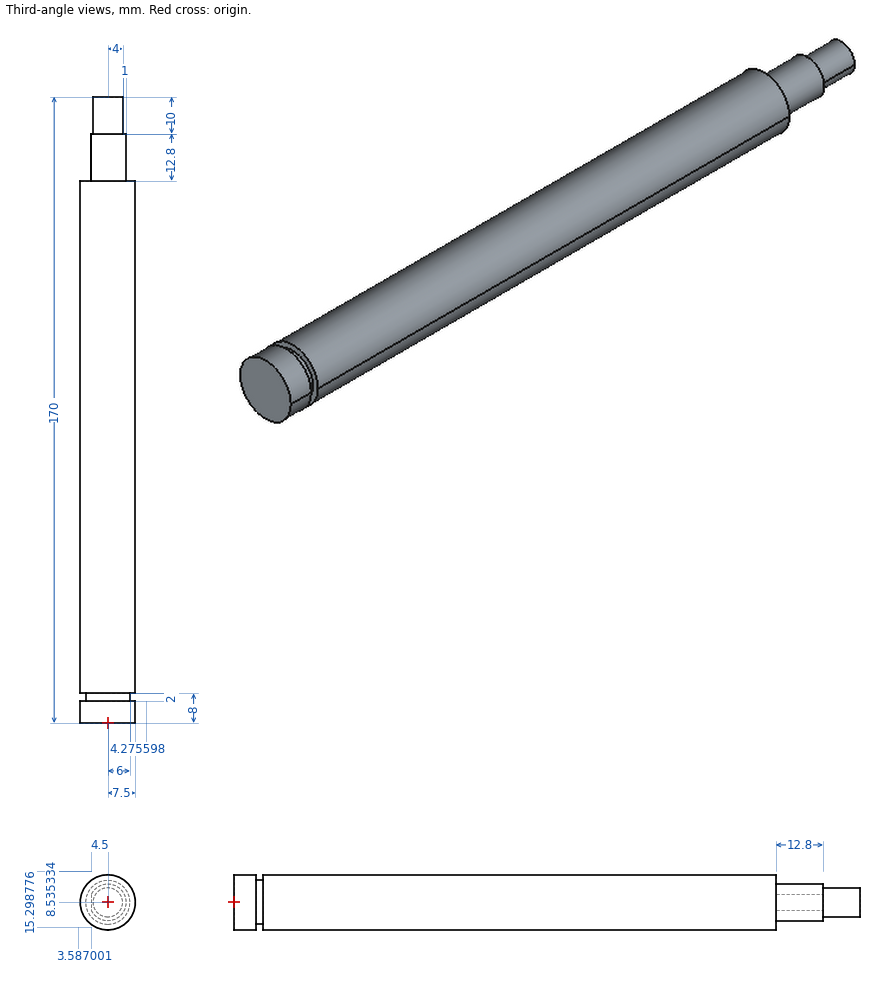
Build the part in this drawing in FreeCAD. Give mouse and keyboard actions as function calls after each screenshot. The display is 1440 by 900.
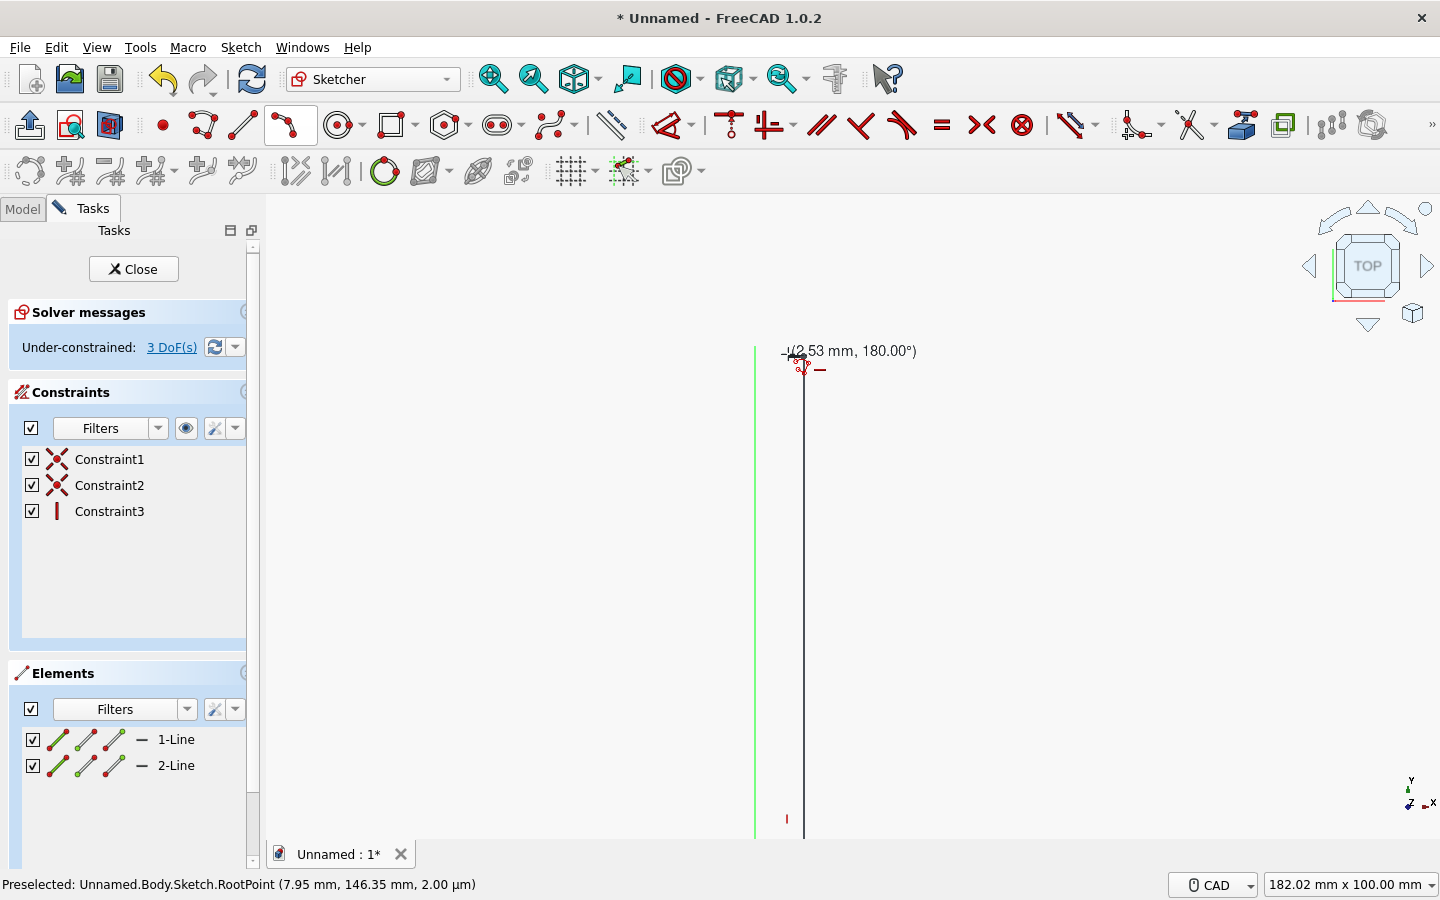
click(787, 354)
click(787, 271)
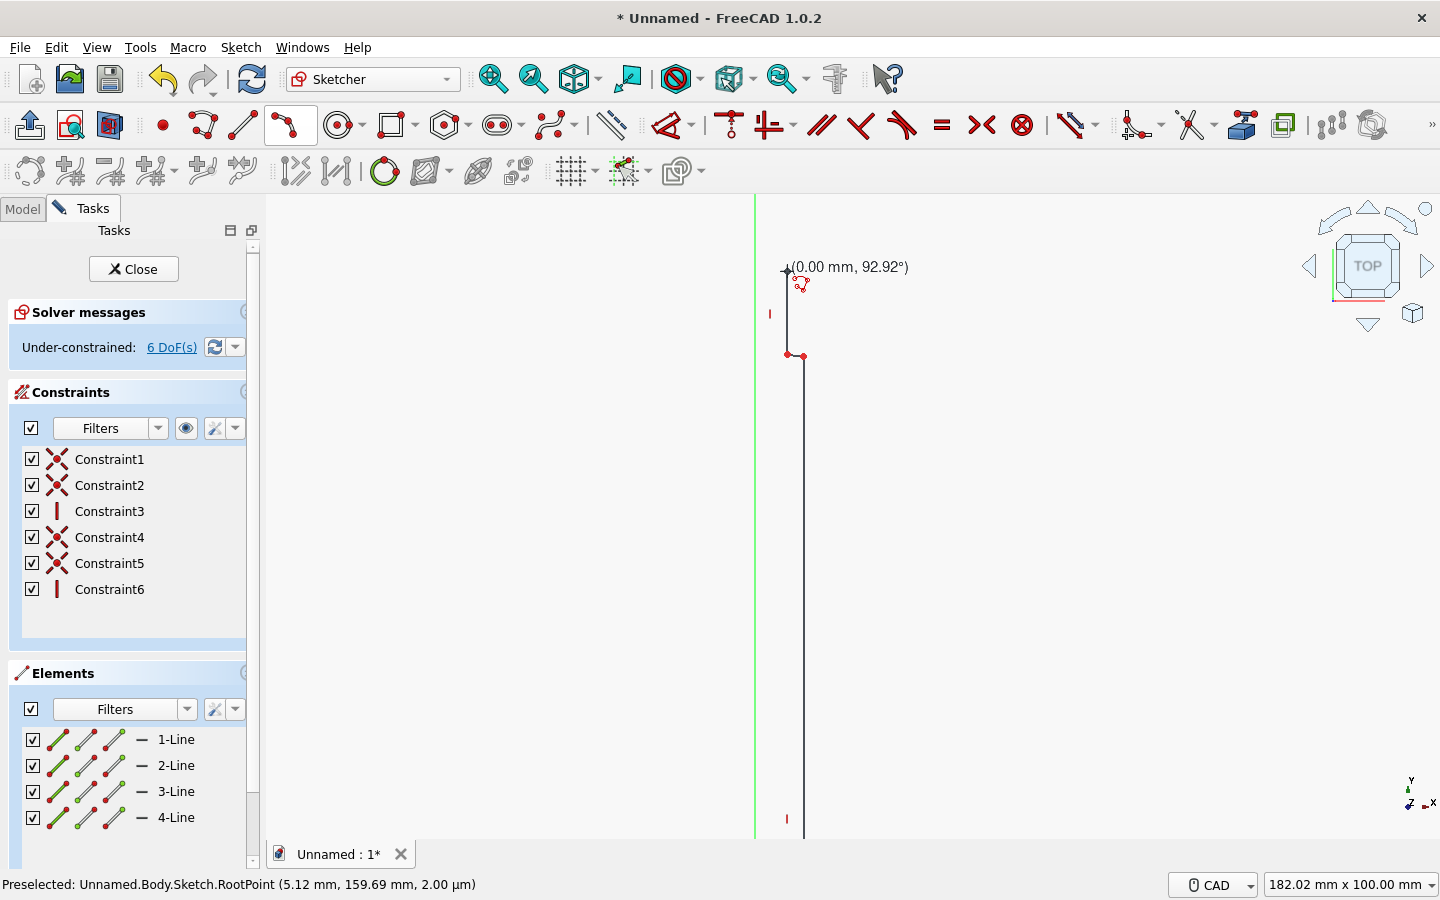
scroll(781, 271, up, 5)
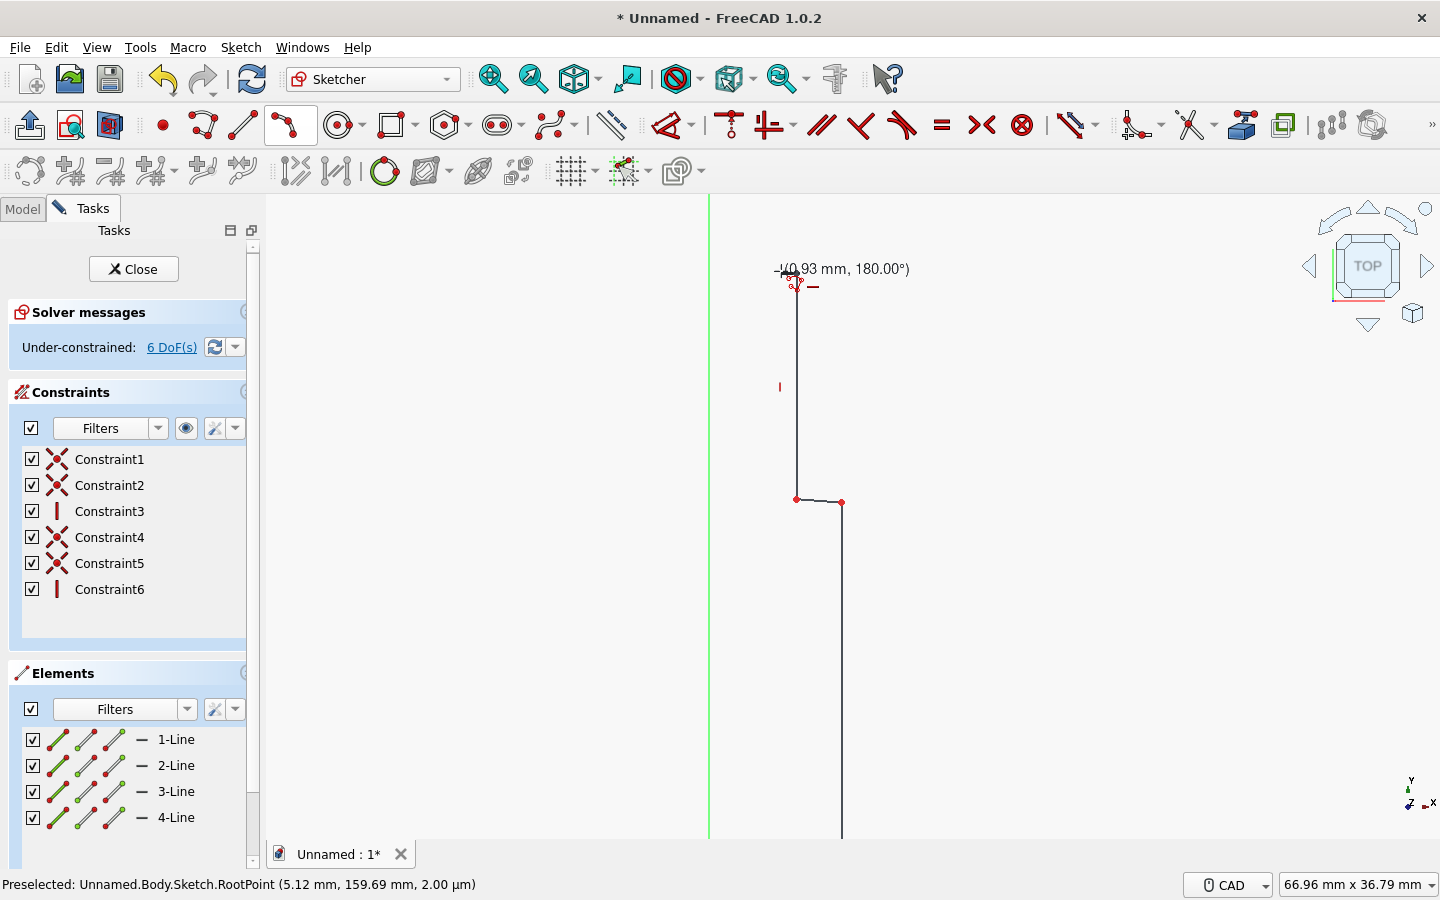
click(780, 271)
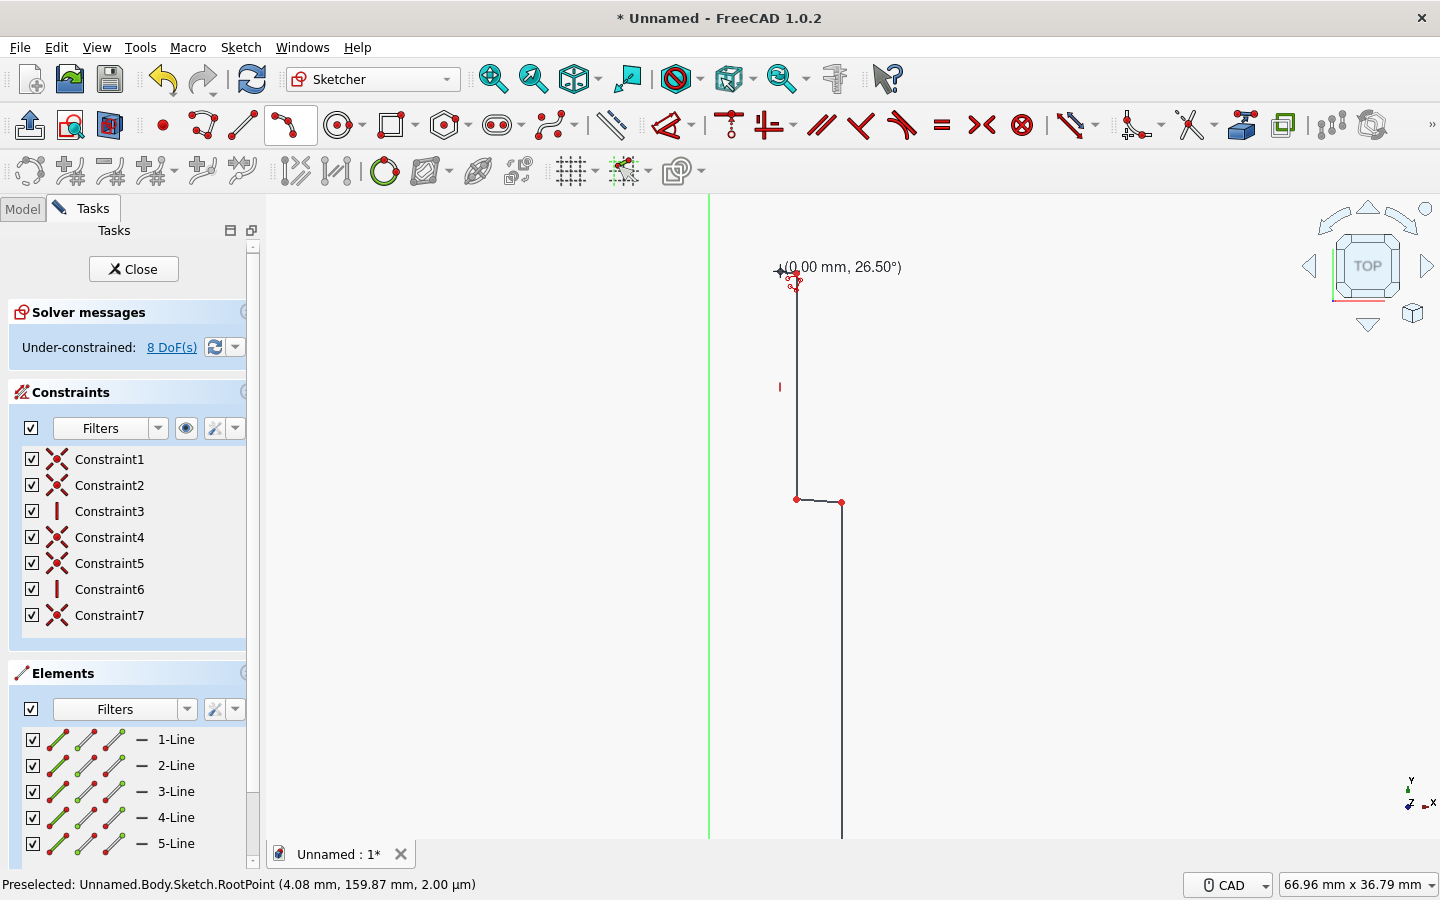
scroll(786, 349, down, 10)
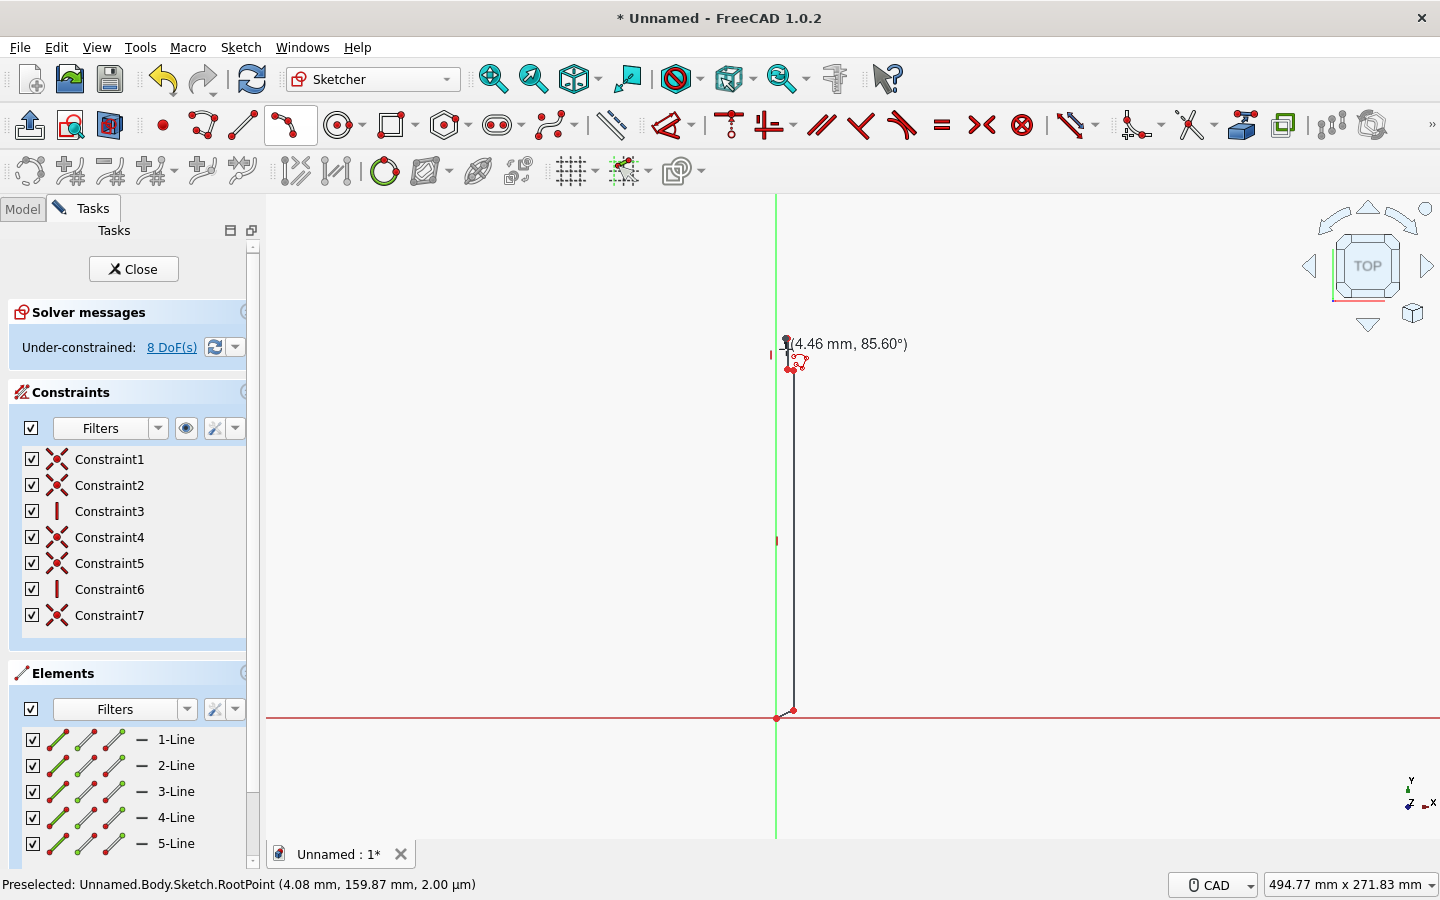
scroll(786, 315, up, 3)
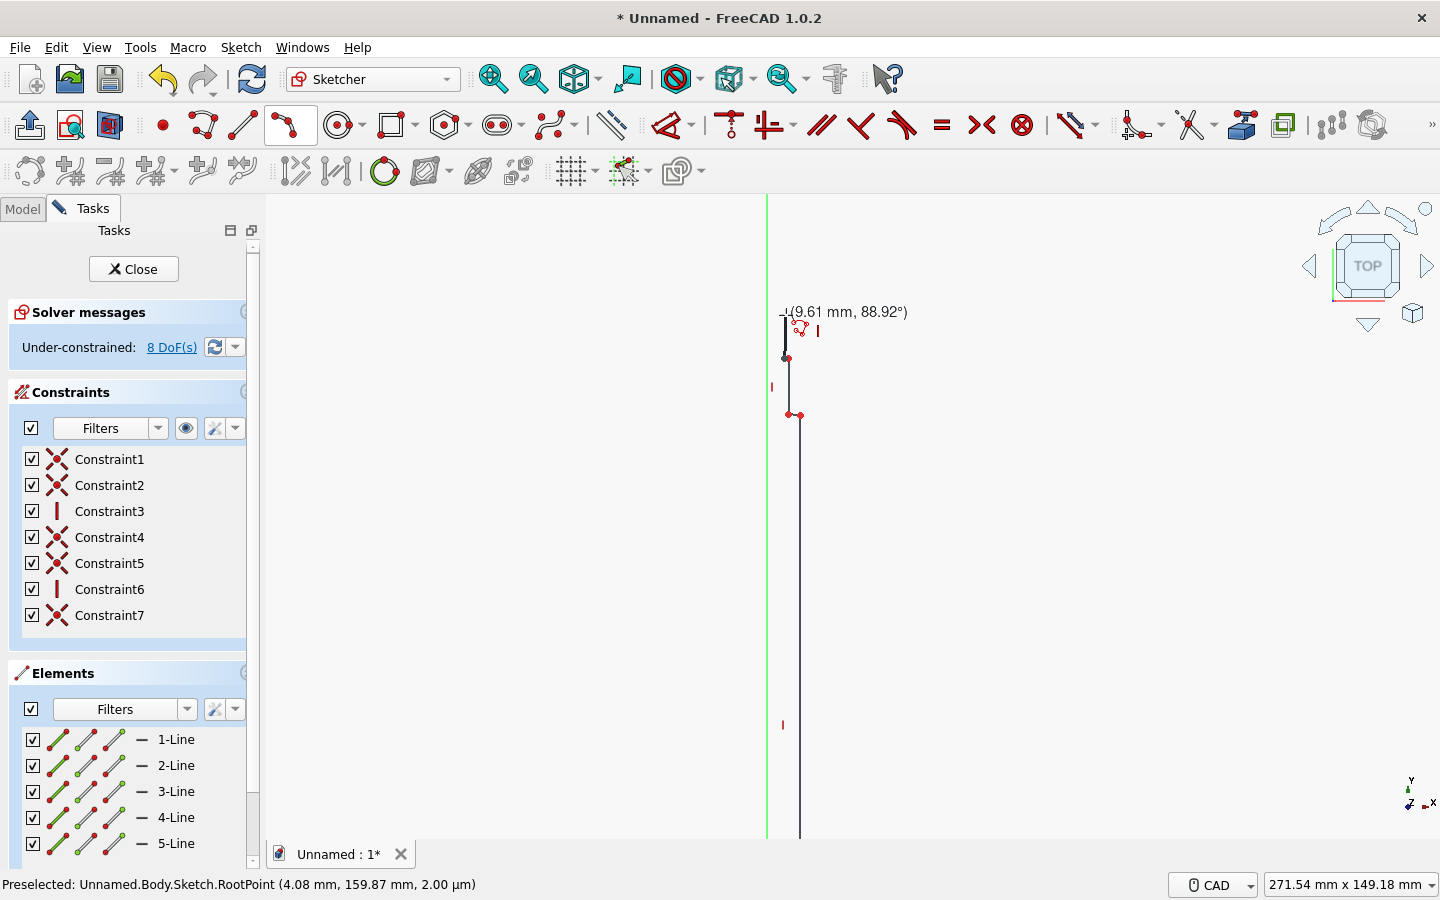
click(785, 315)
click(776, 315)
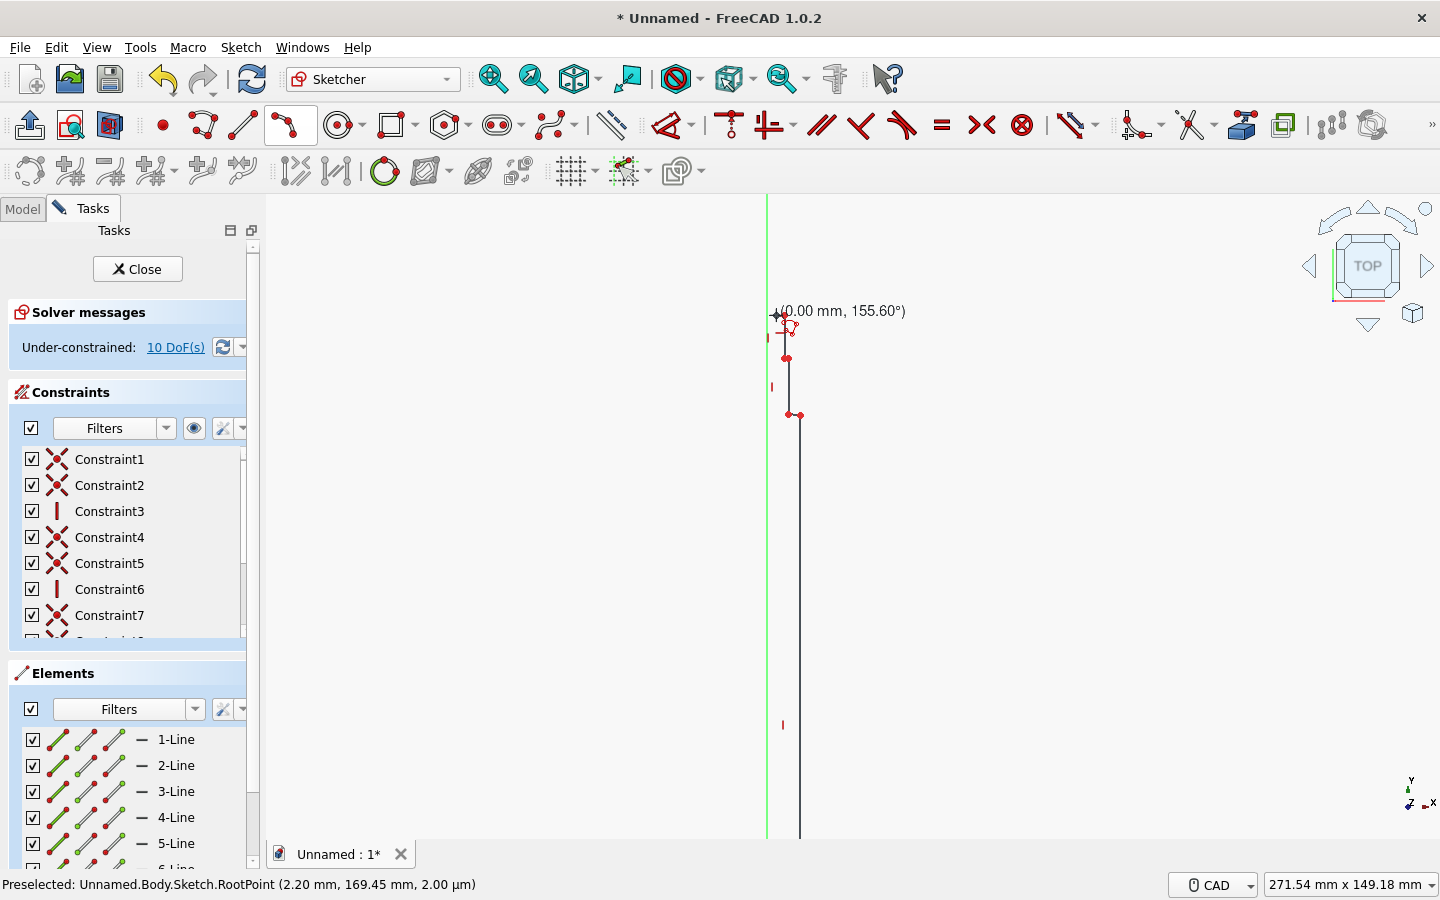
scroll(785, 315, down, 3)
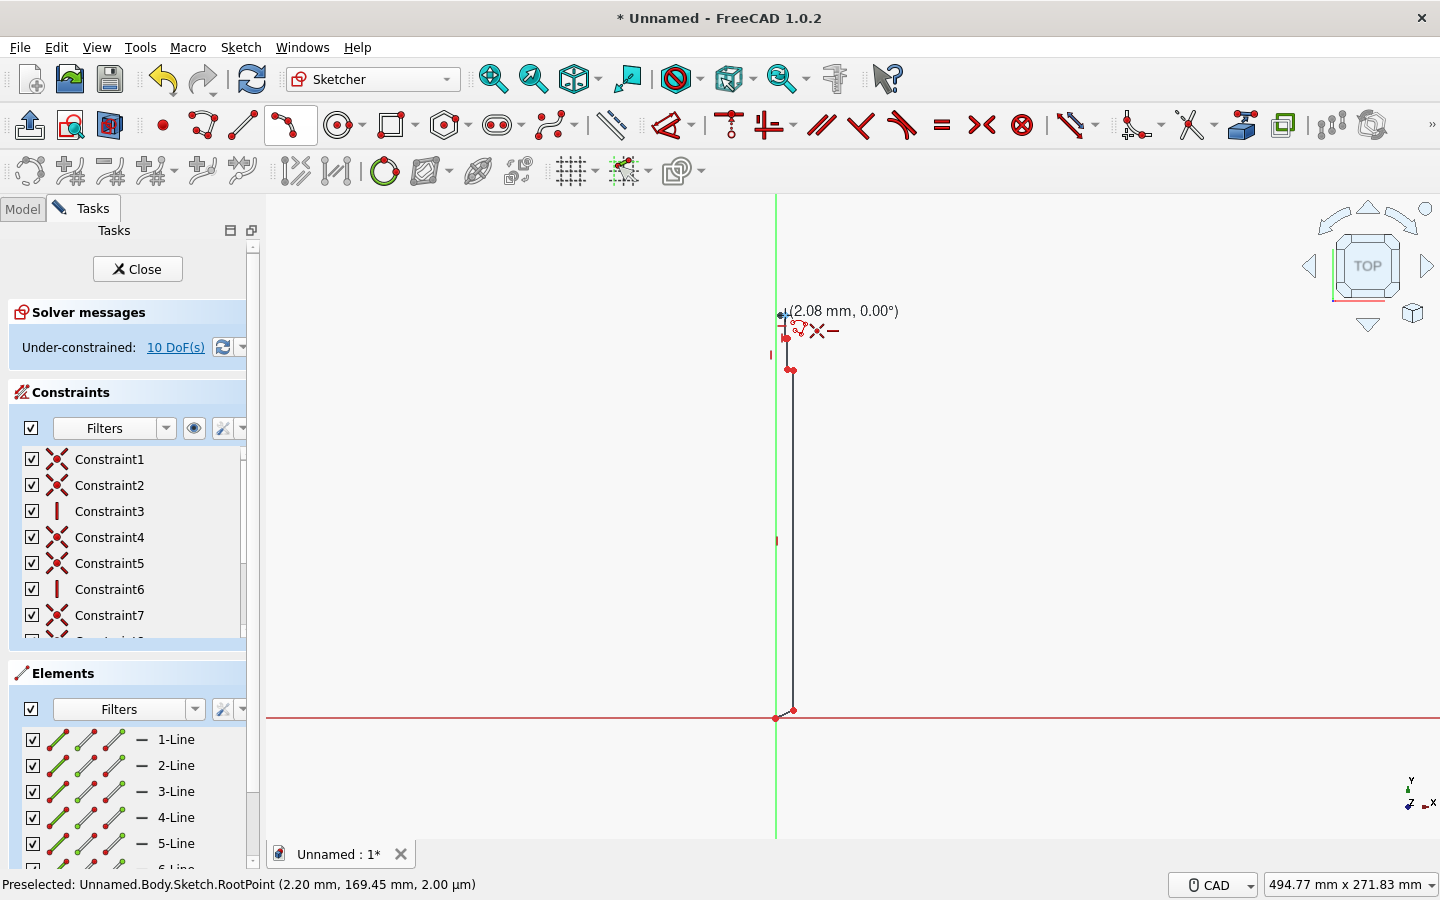
scroll(776, 718, up, 3)